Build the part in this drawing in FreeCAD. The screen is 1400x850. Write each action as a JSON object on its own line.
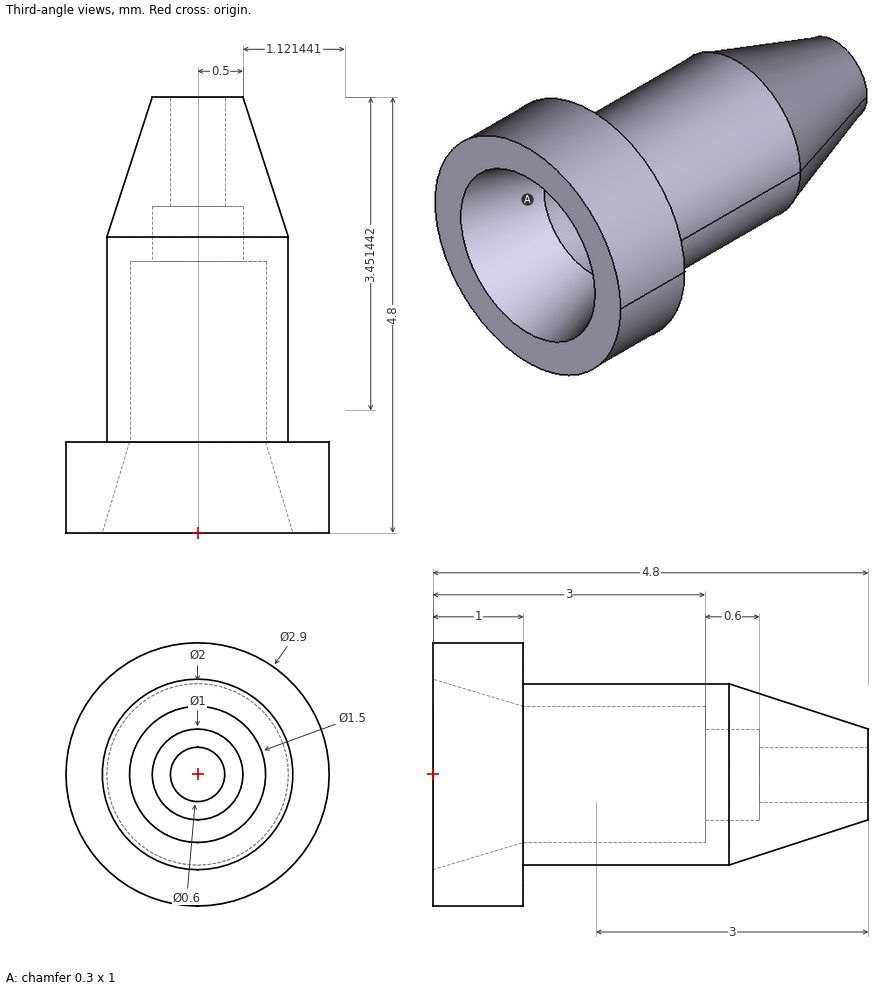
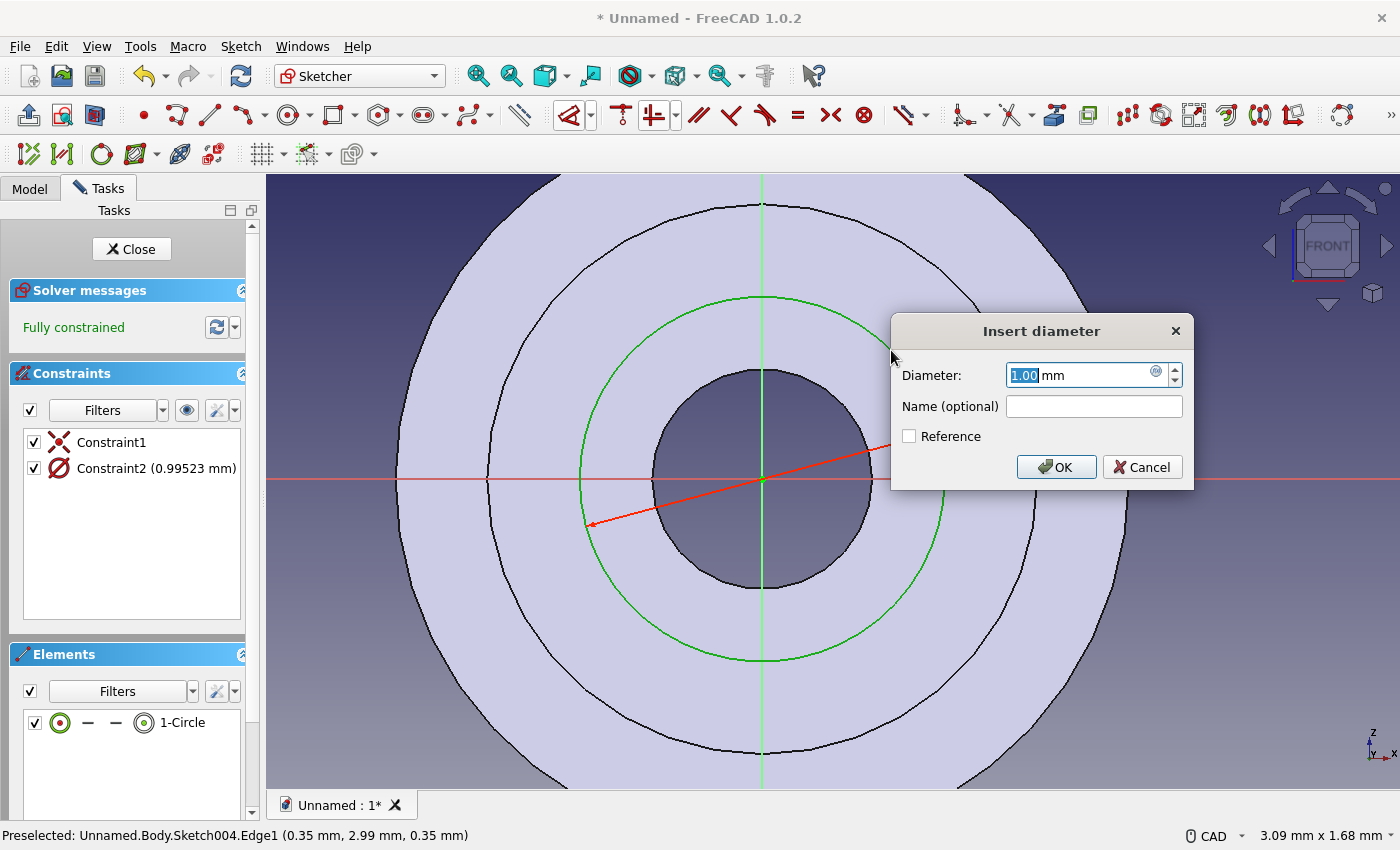
{"action": "type", "text": "1"}
{"action": "key", "text": "Return"}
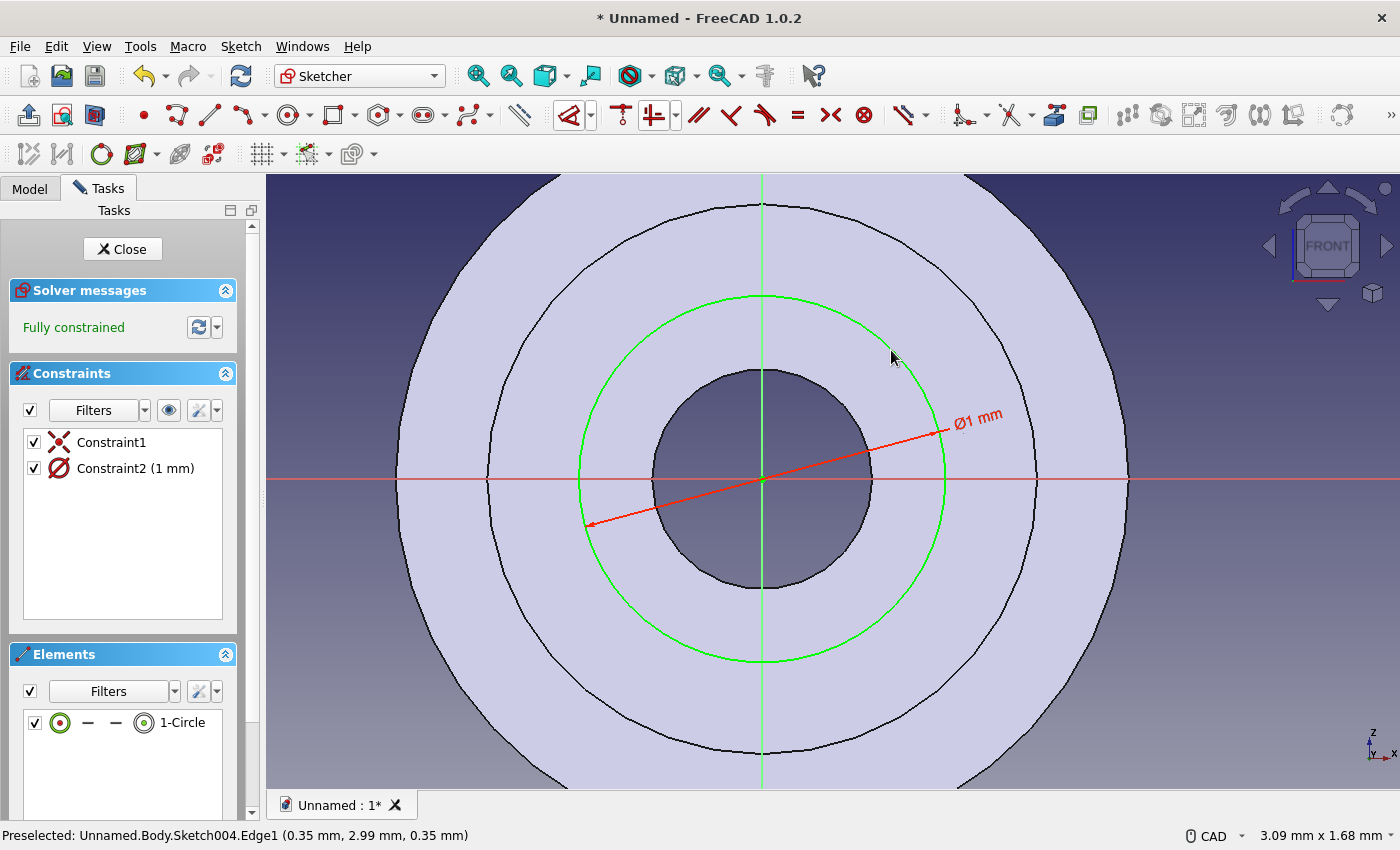
{"action": "left_click", "coordinate": [123, 249]}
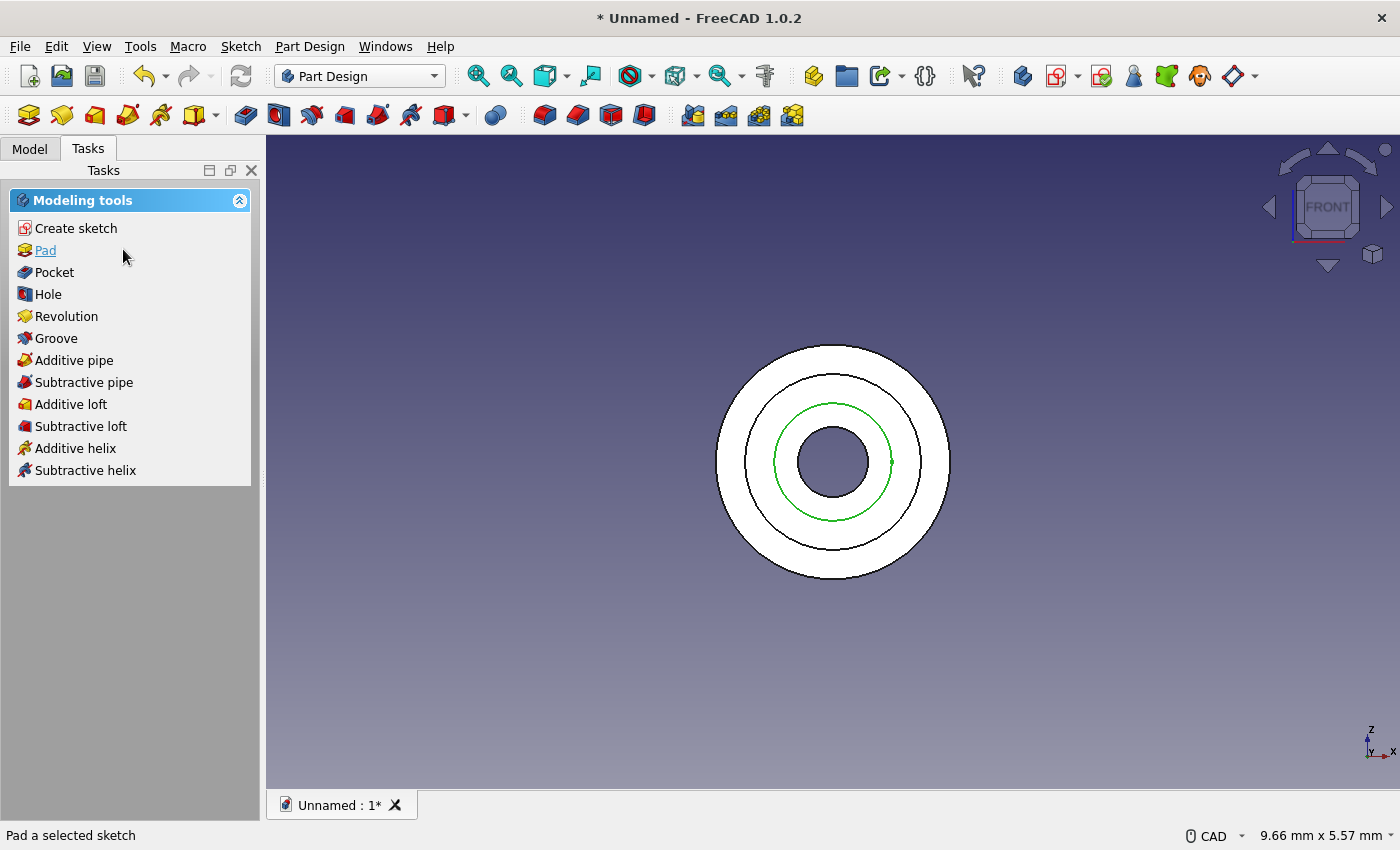
{"action": "left_click", "coordinate": [246, 116]}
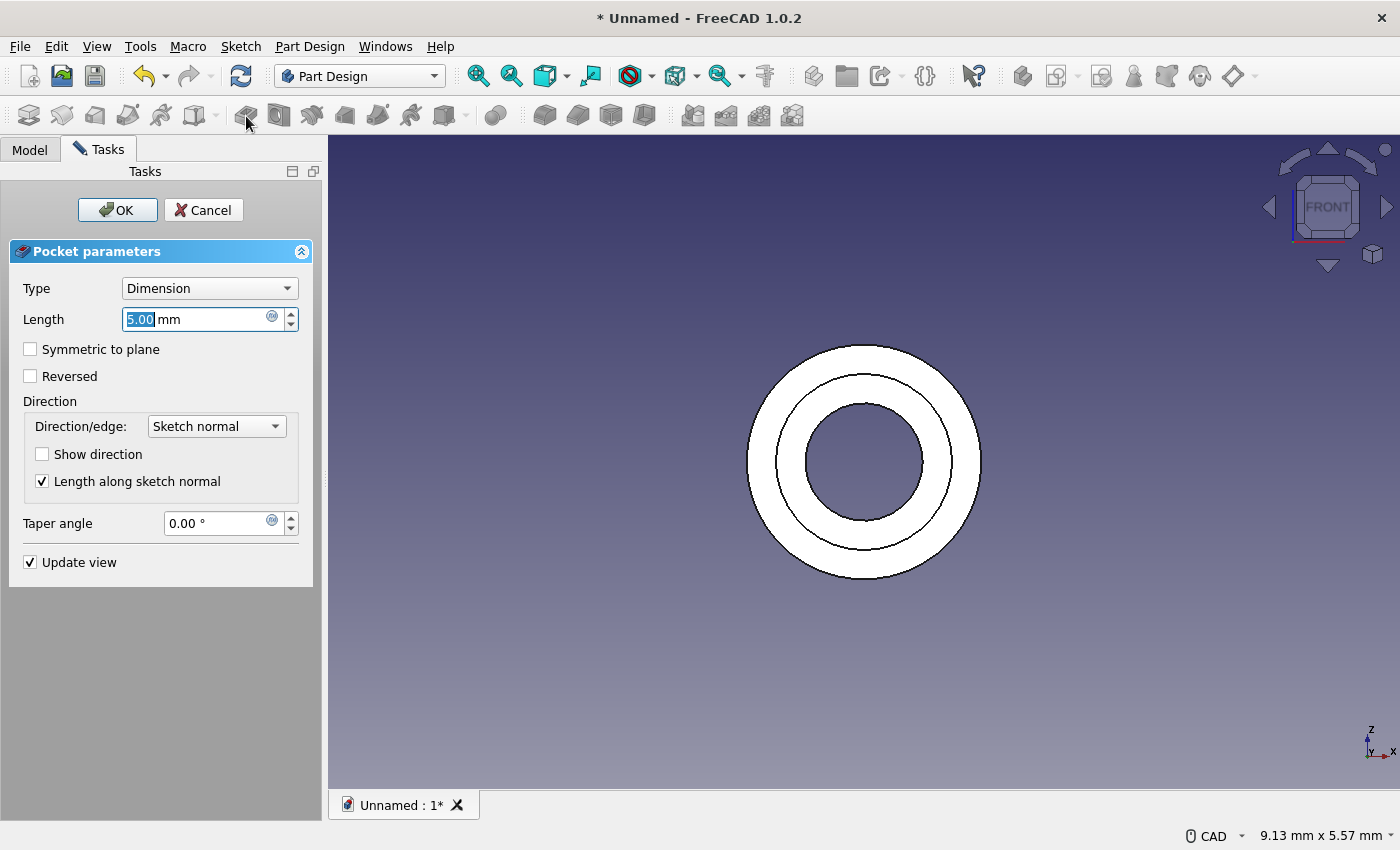
{"action": "type", "text": "0.6"}
{"action": "key", "text": "Tab"}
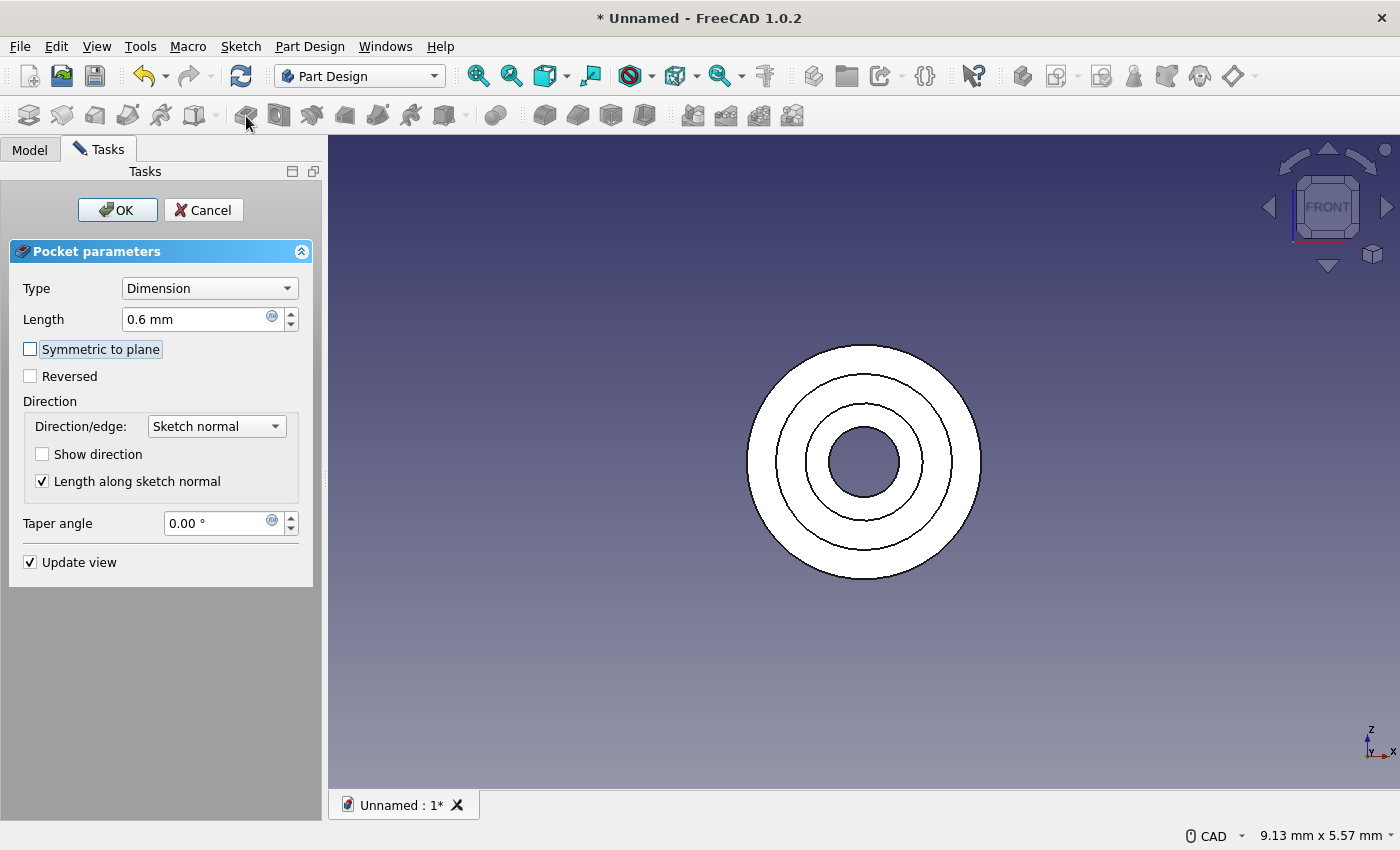
{"action": "left_click", "coordinate": [118, 210]}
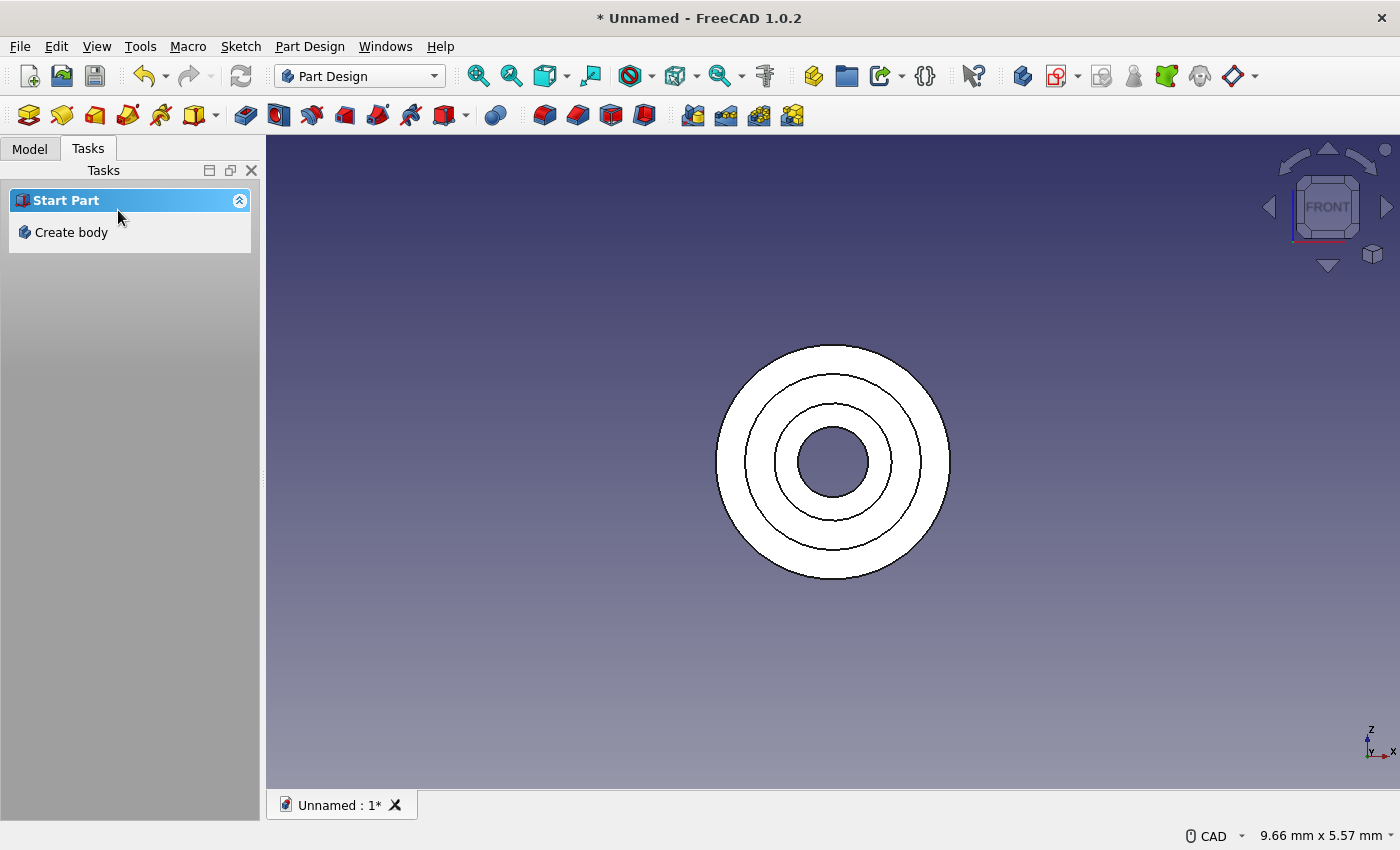
{"action": "left_click", "coordinate": [479, 76]}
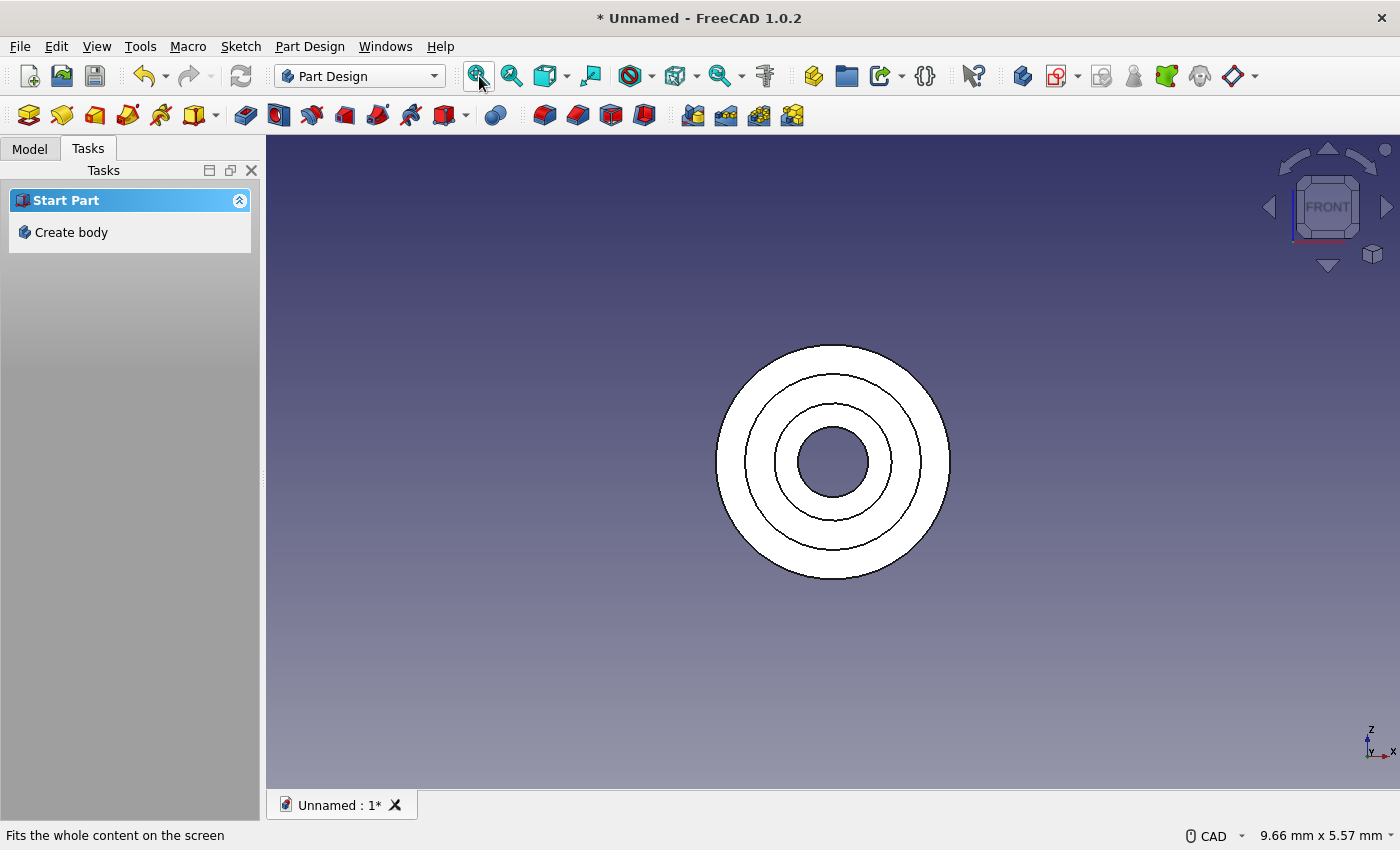
{"action": "left_click", "coordinate": [1056, 76]}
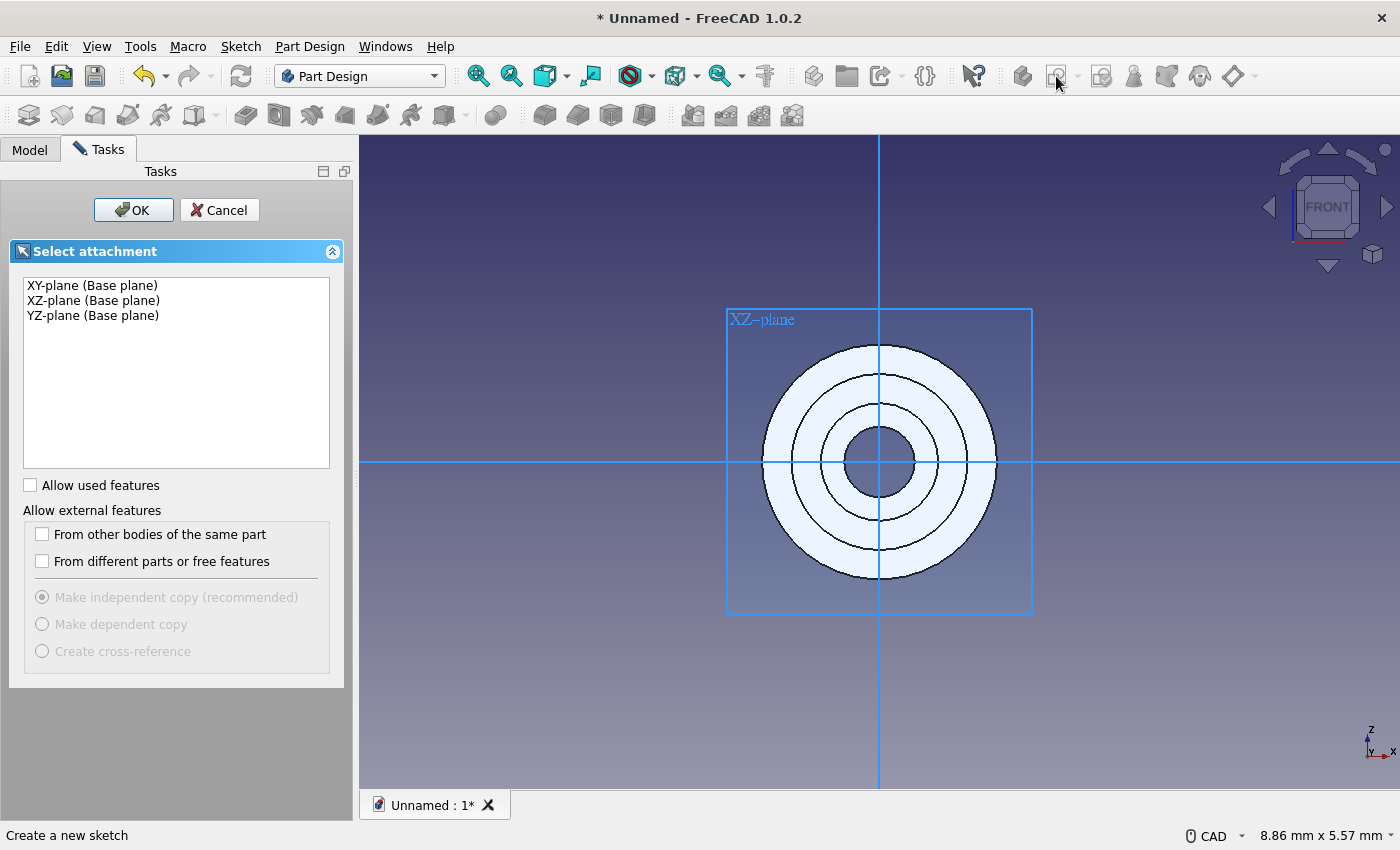
{"action": "left_click", "coordinate": [84, 300]}